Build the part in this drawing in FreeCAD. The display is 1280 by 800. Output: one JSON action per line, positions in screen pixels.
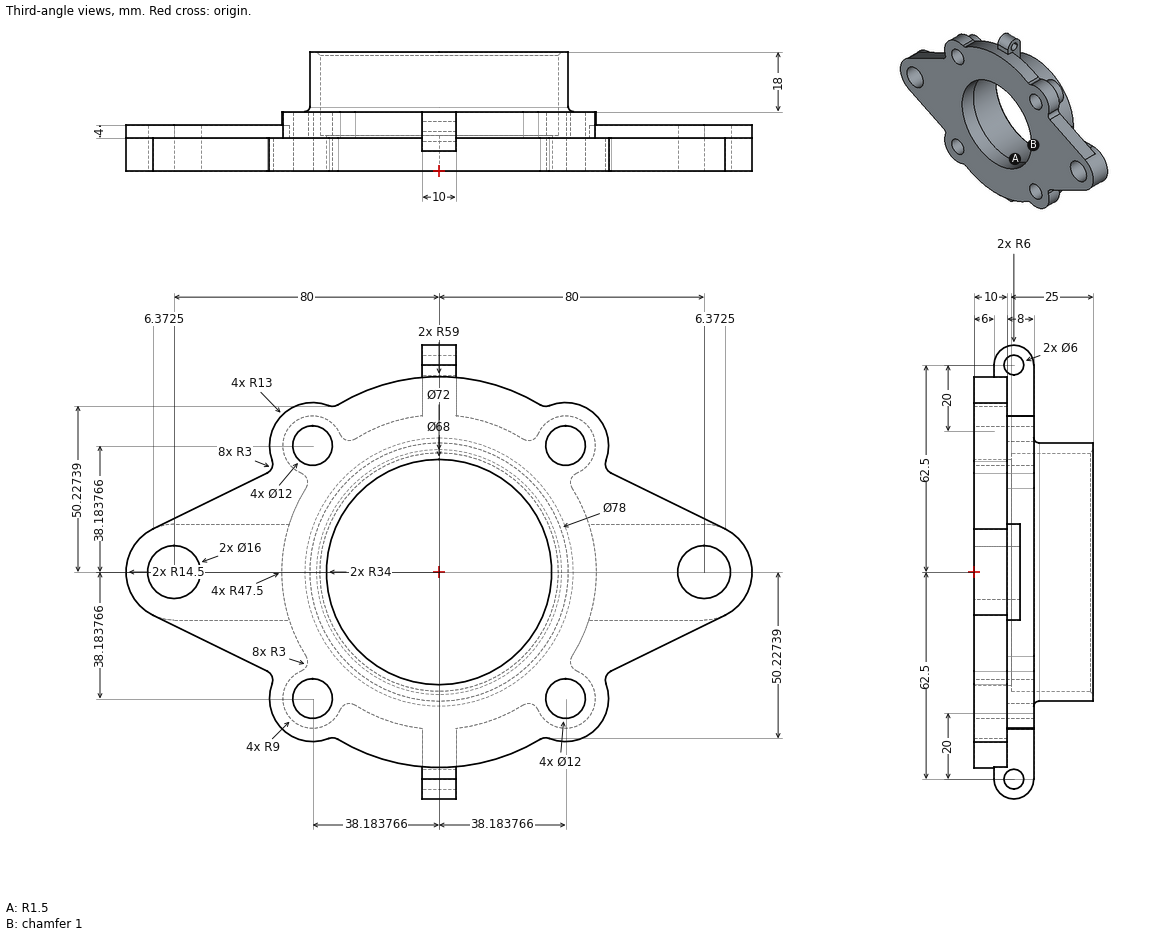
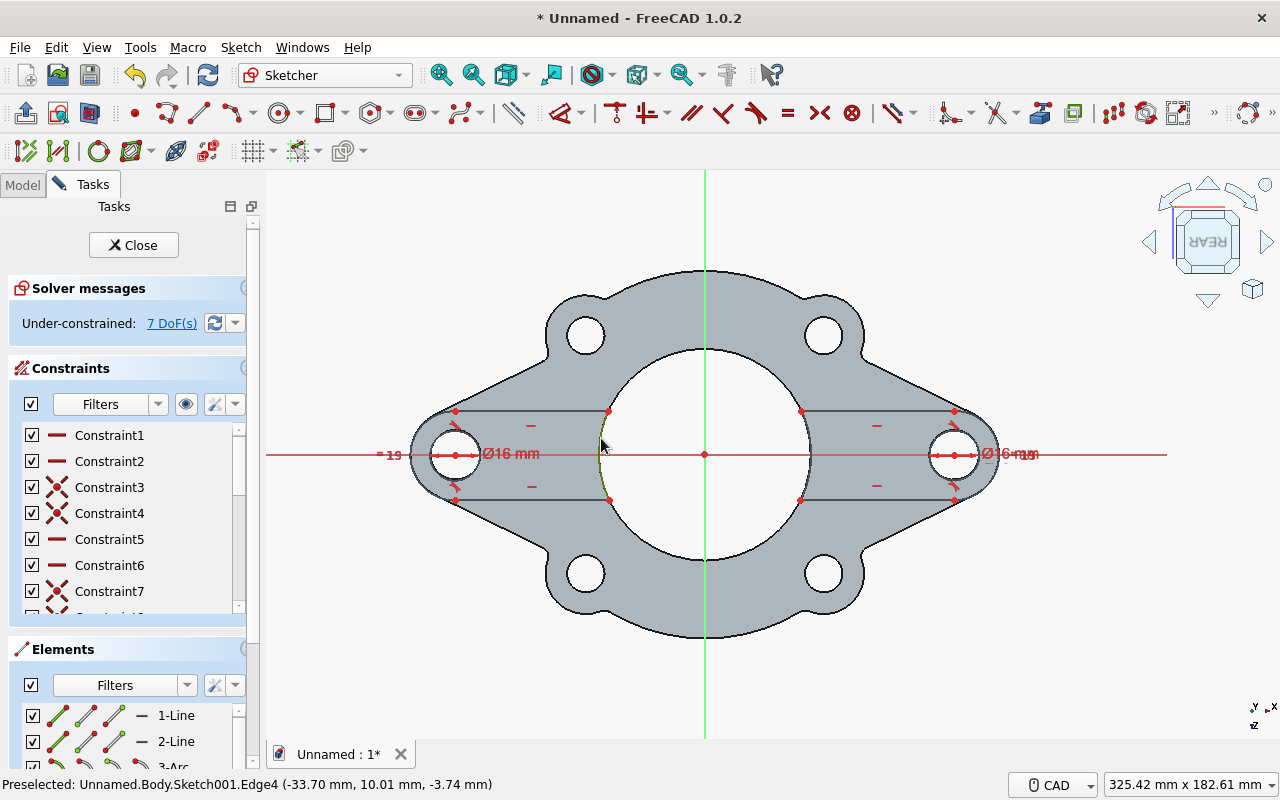
{"action": "left_click", "coordinate": [809, 474]}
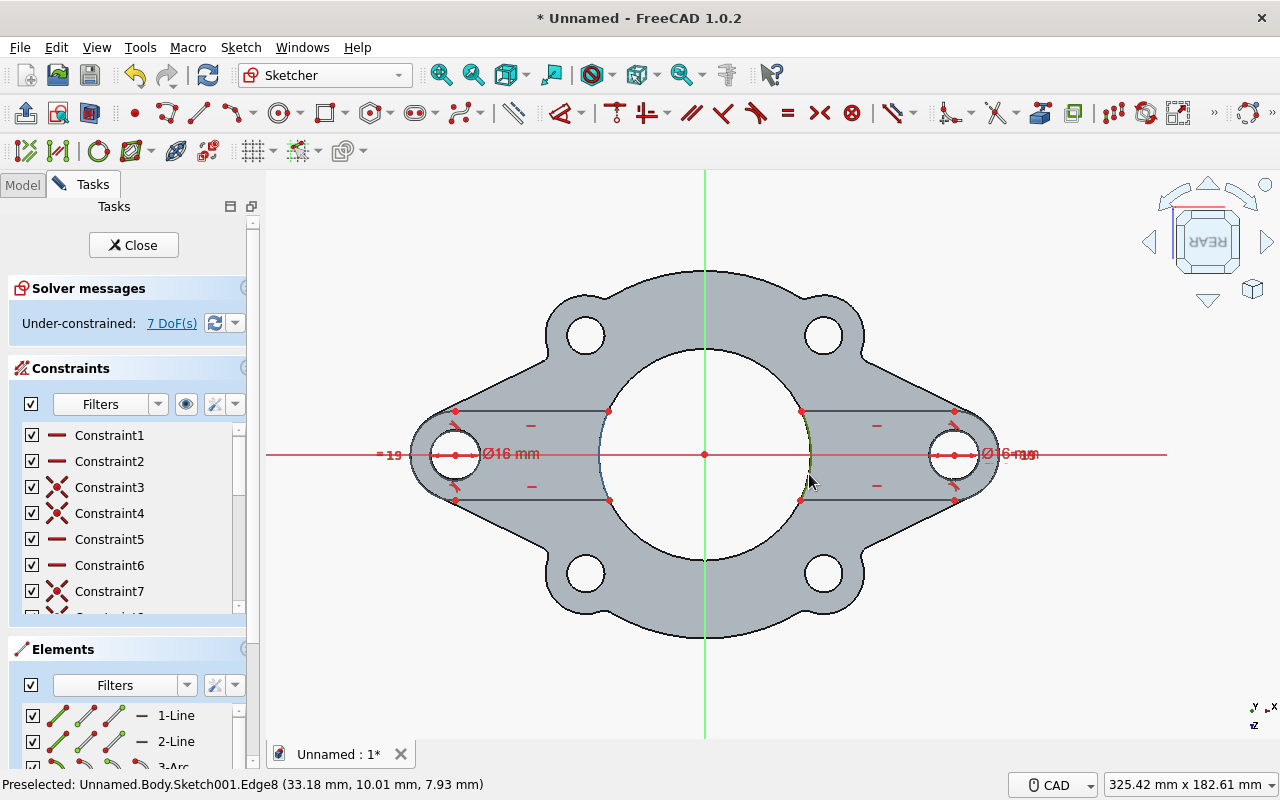
{"action": "left_click", "coordinate": [788, 114]}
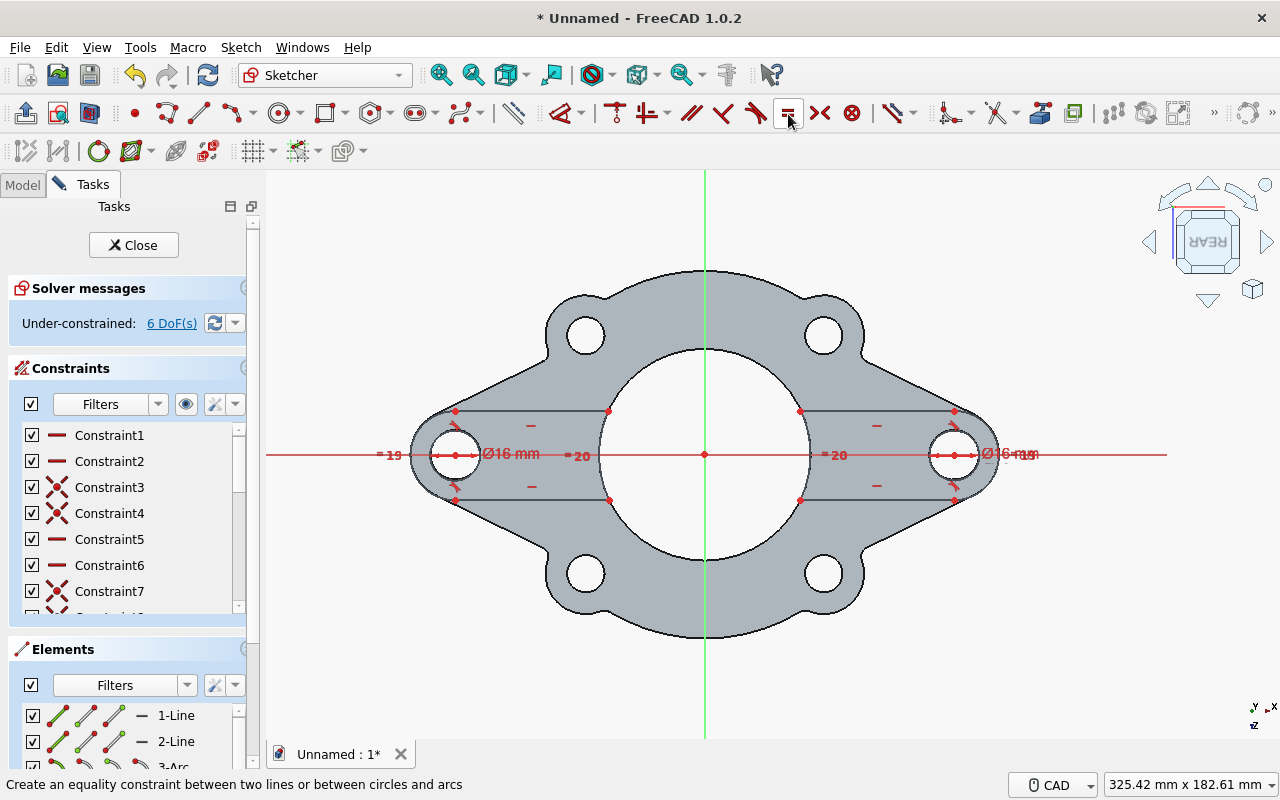
{"action": "left_click", "coordinate": [455, 456]}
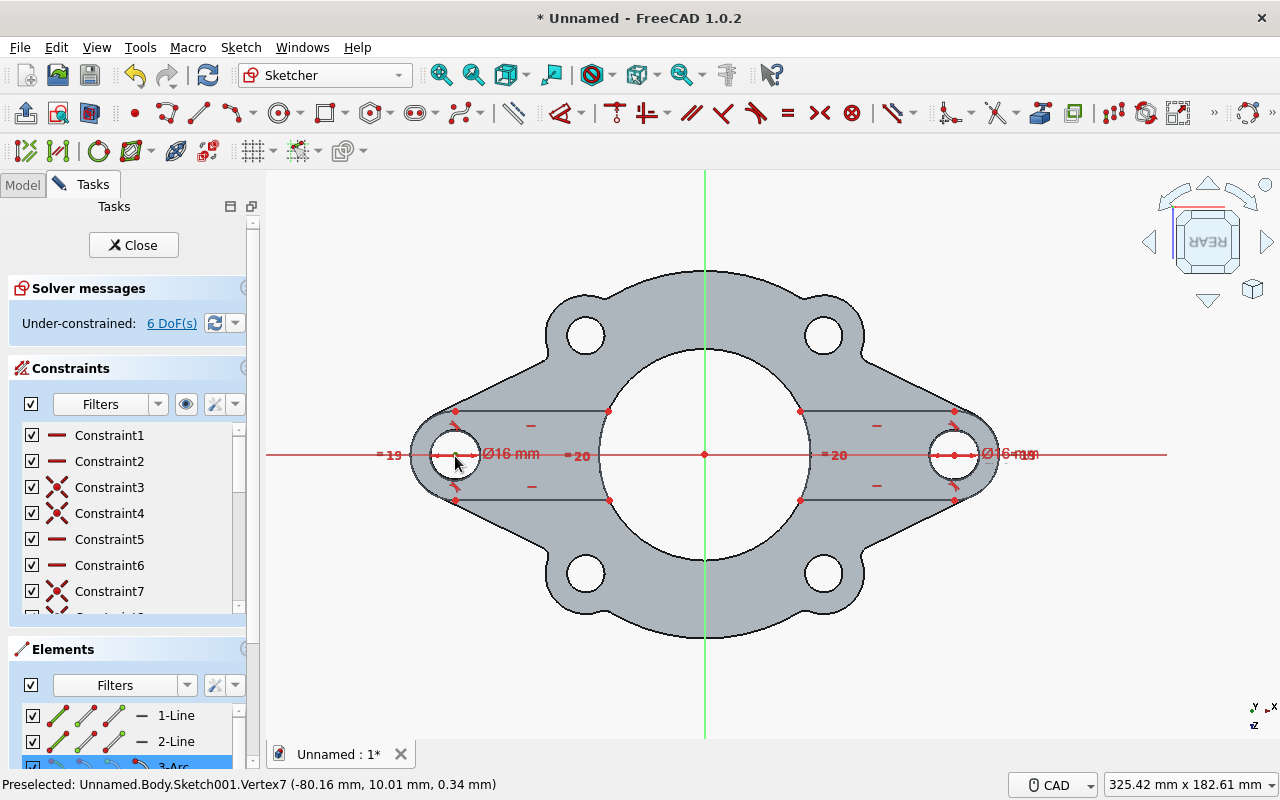
{"action": "left_click", "coordinate": [353, 455]}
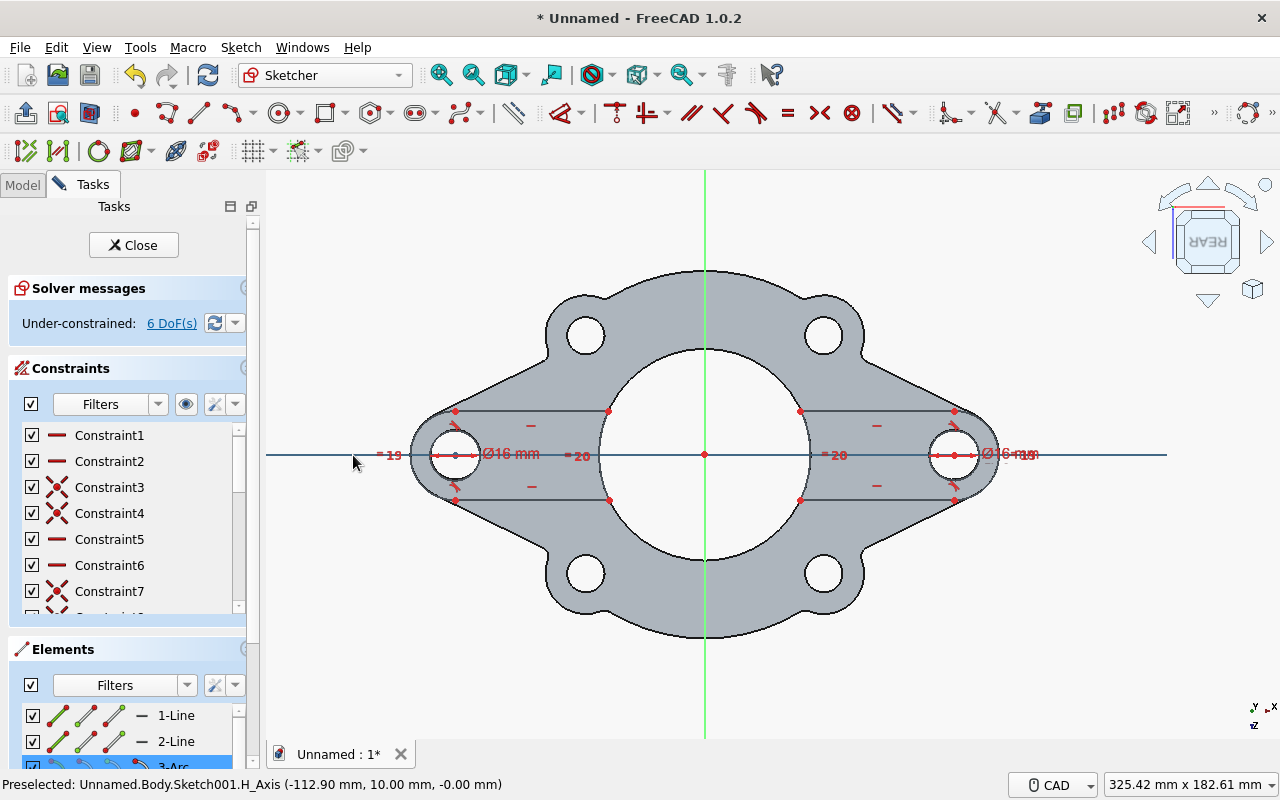
{"action": "left_click", "coordinate": [616, 114]}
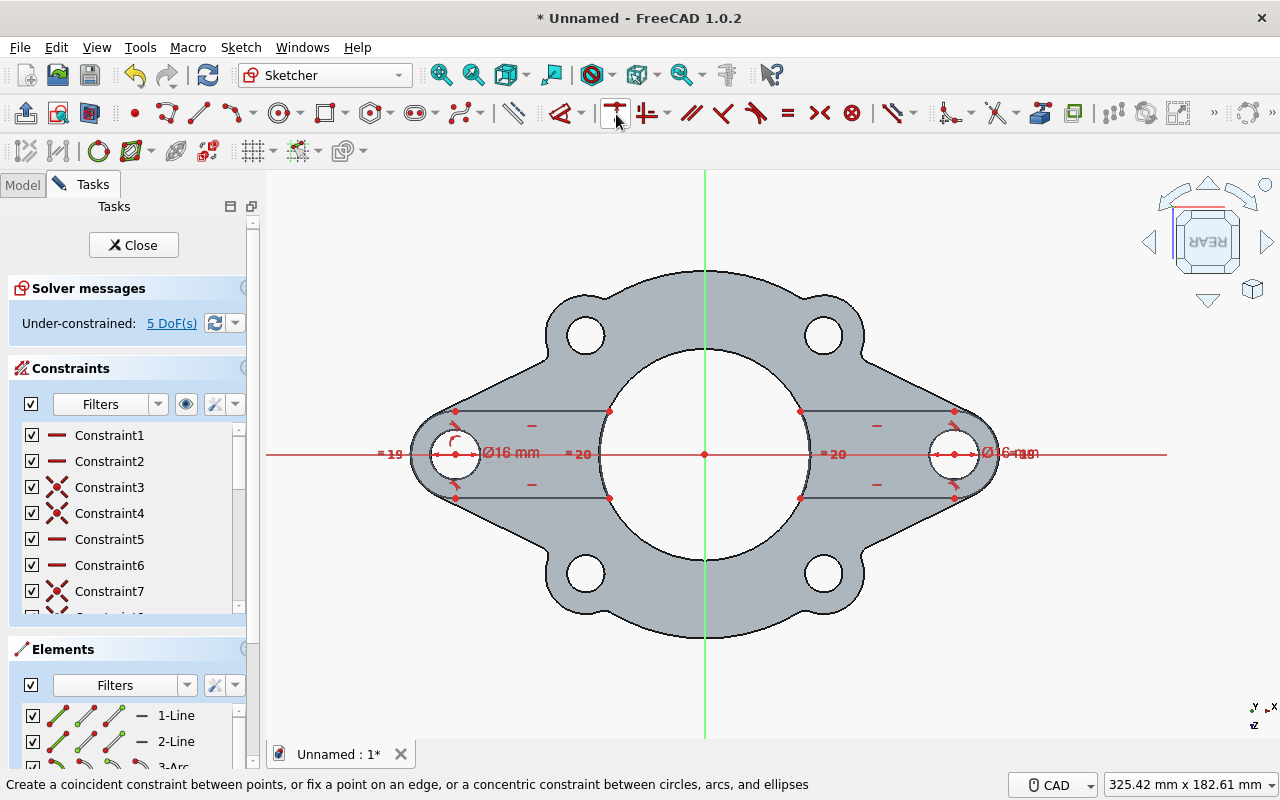
{"action": "left_click", "coordinate": [954, 455]}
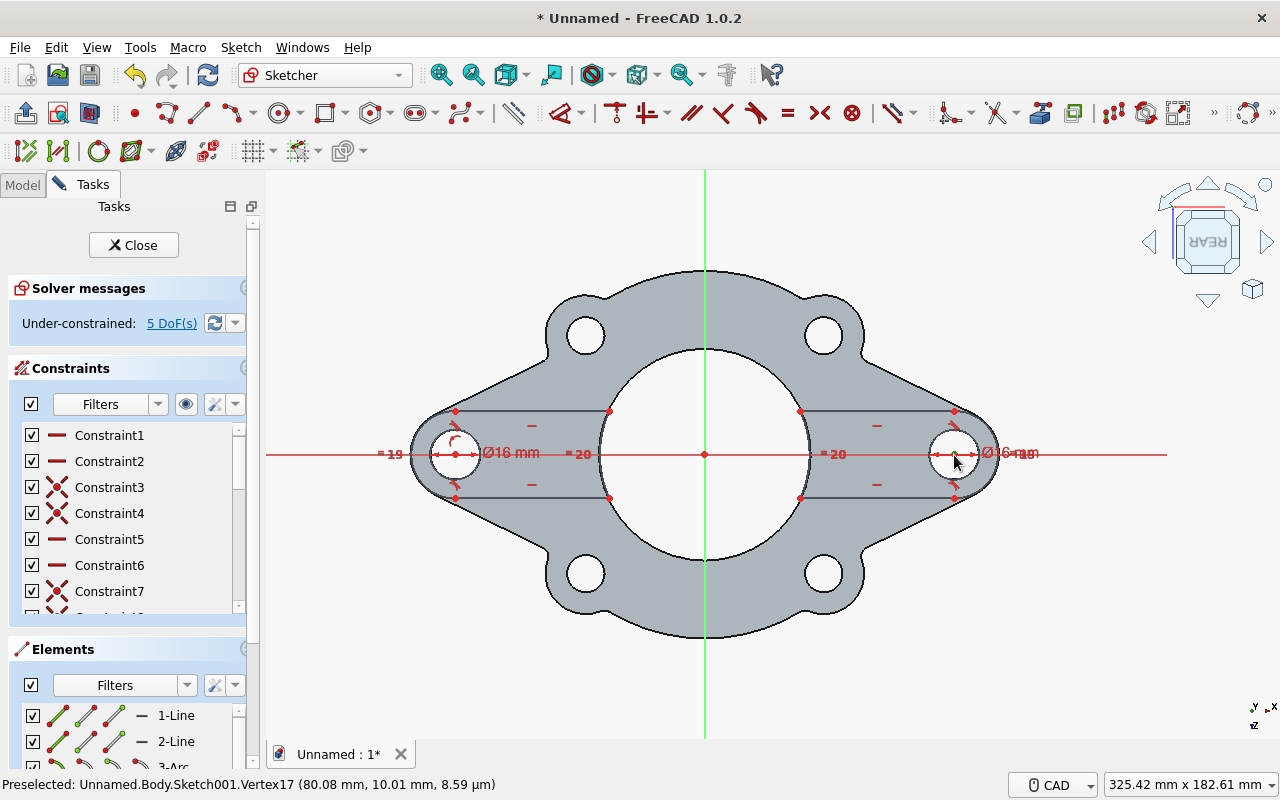
{"action": "left_click", "coordinate": [353, 455]}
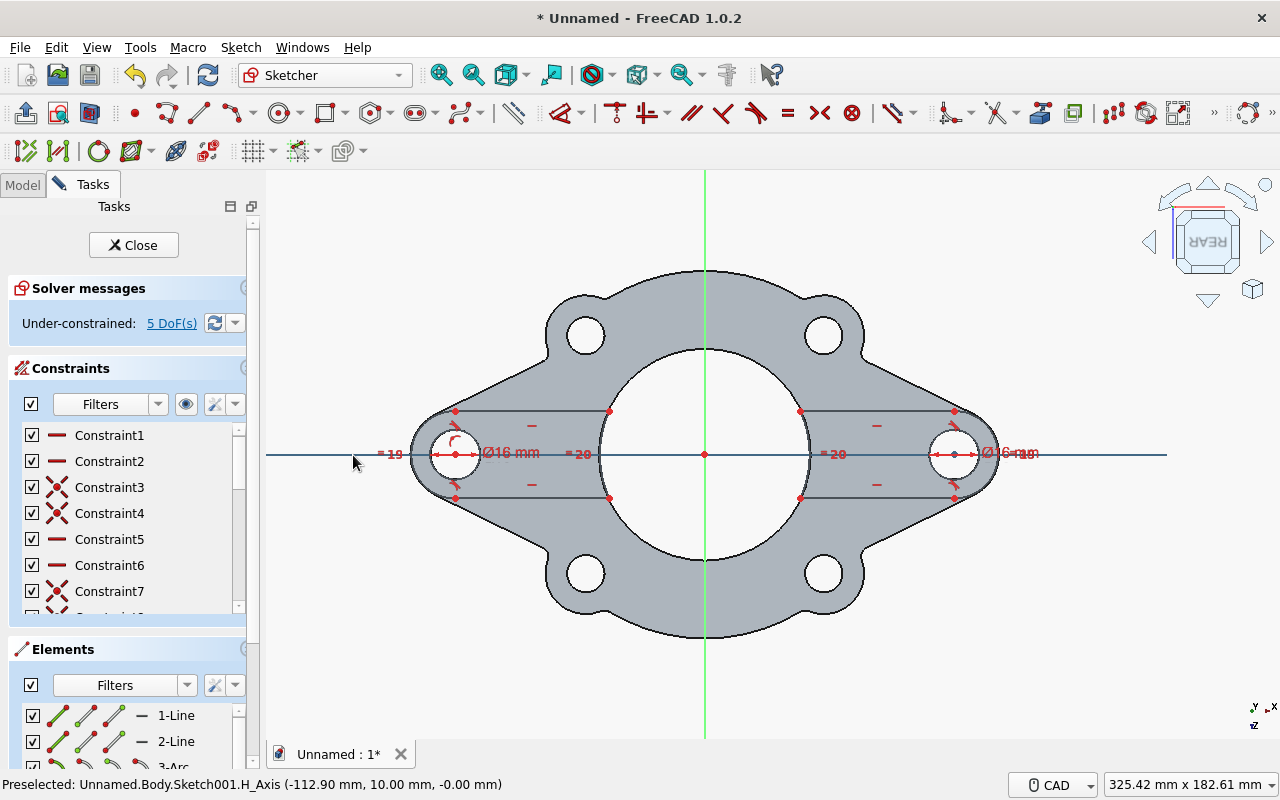
{"action": "left_click", "coordinate": [616, 114]}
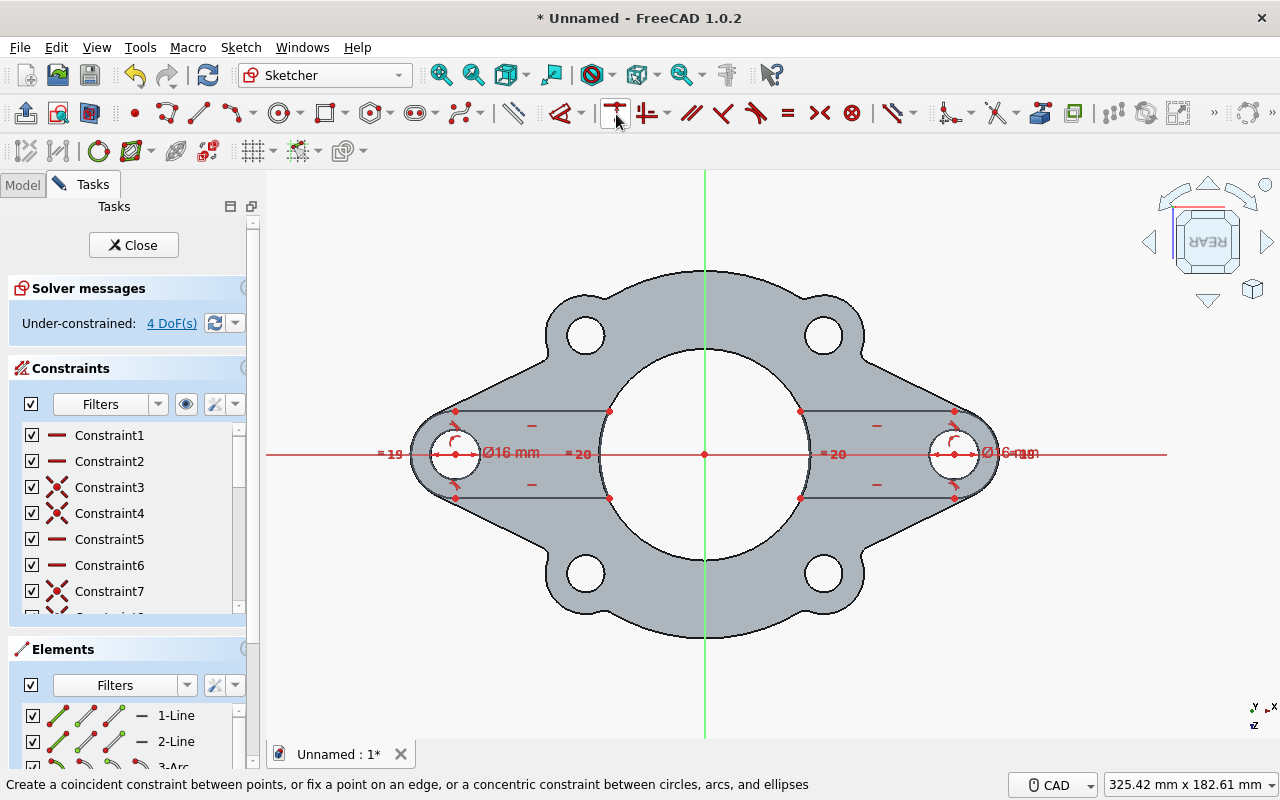
{"action": "left_click", "coordinate": [560, 114]}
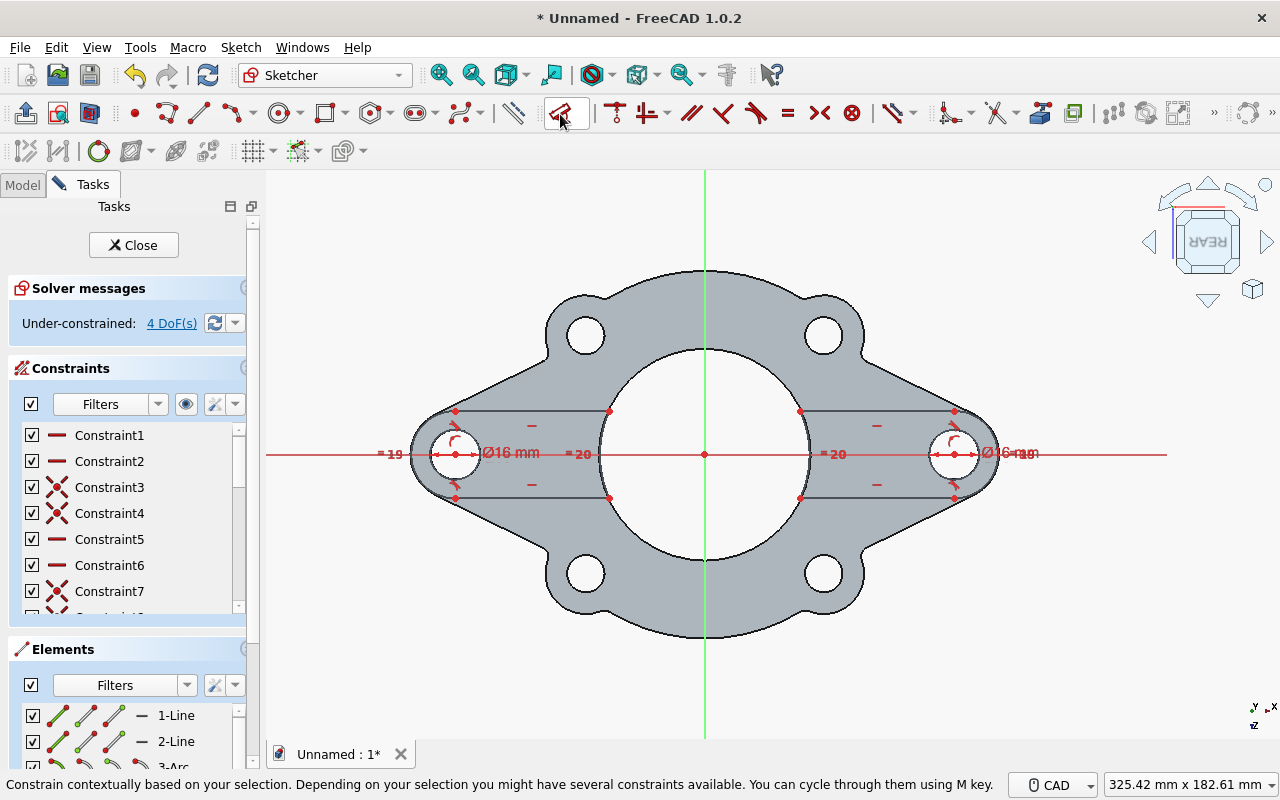
{"action": "left_click", "coordinate": [420, 429]}
{"action": "left_click", "coordinate": [394, 410]}